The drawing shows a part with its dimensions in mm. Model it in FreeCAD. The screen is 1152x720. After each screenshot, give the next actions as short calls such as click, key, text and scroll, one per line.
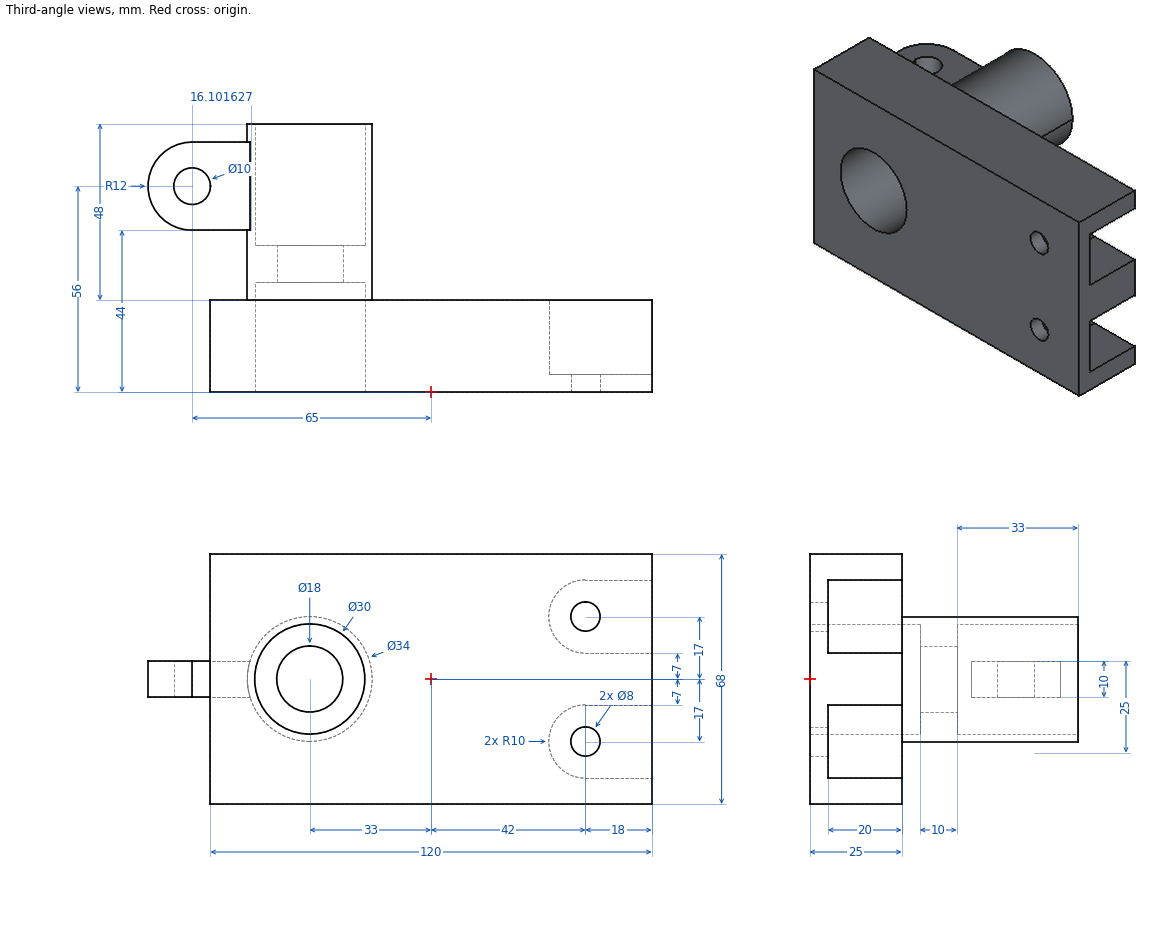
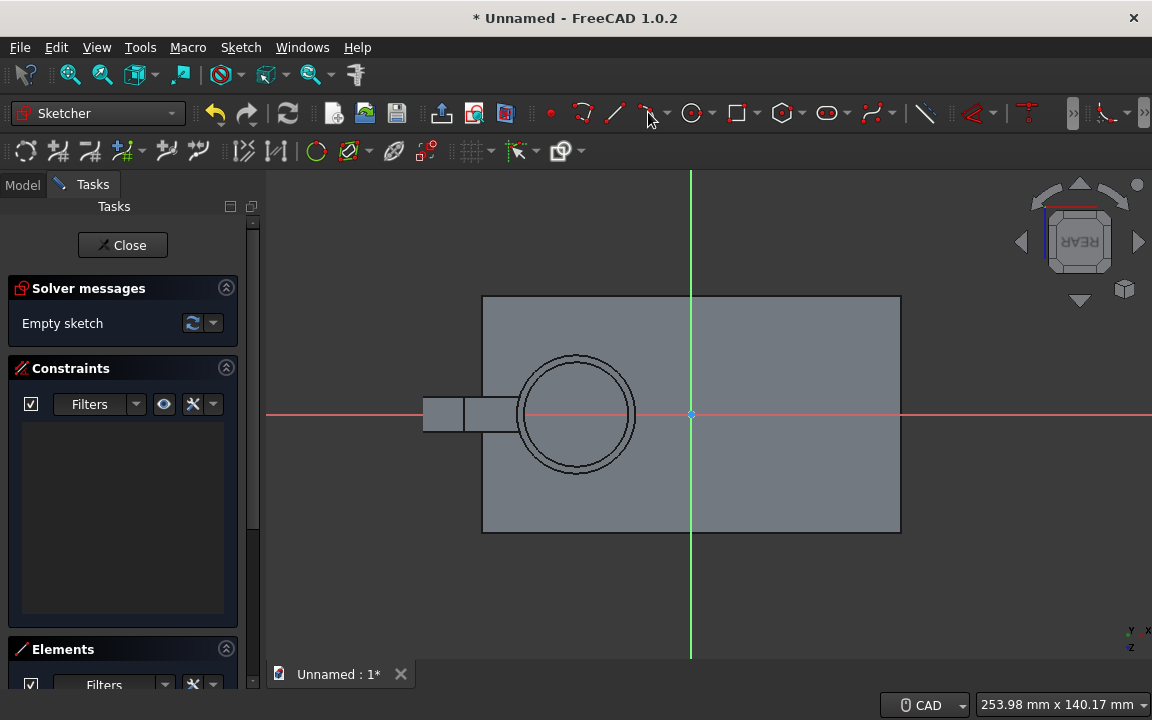
scroll(608, 414, up, 6)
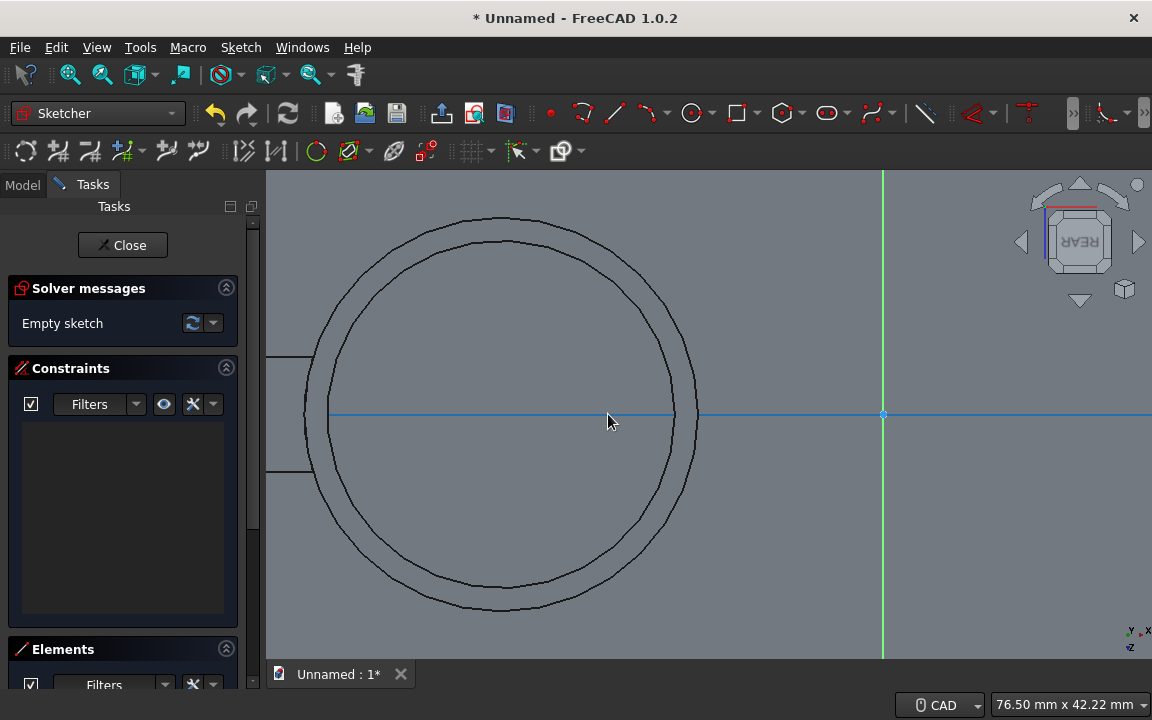
click(692, 114)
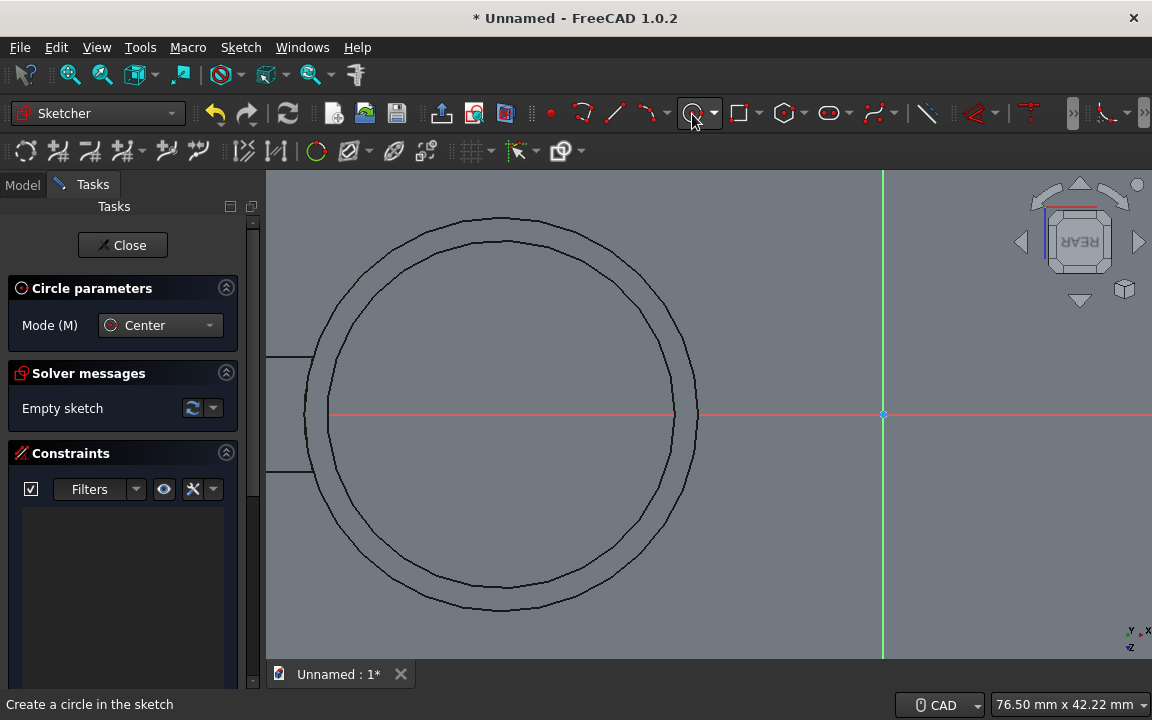
click(501, 414)
move(575, 341)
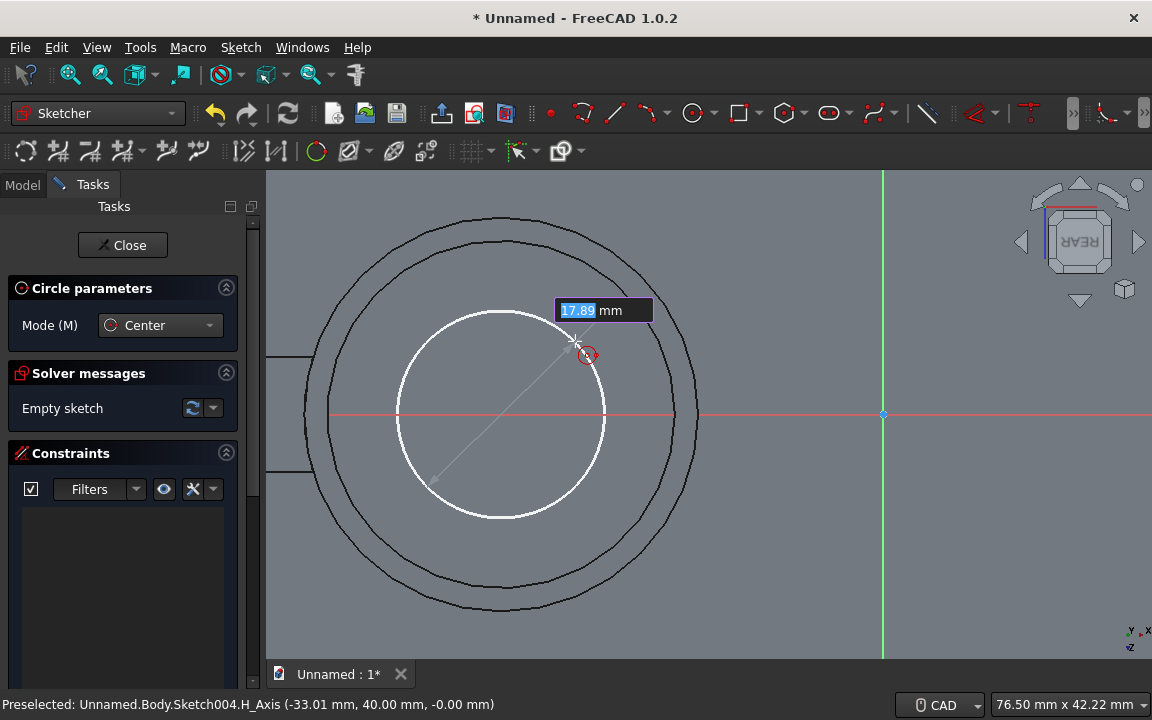
text(18)
key(Return)
key(Escape)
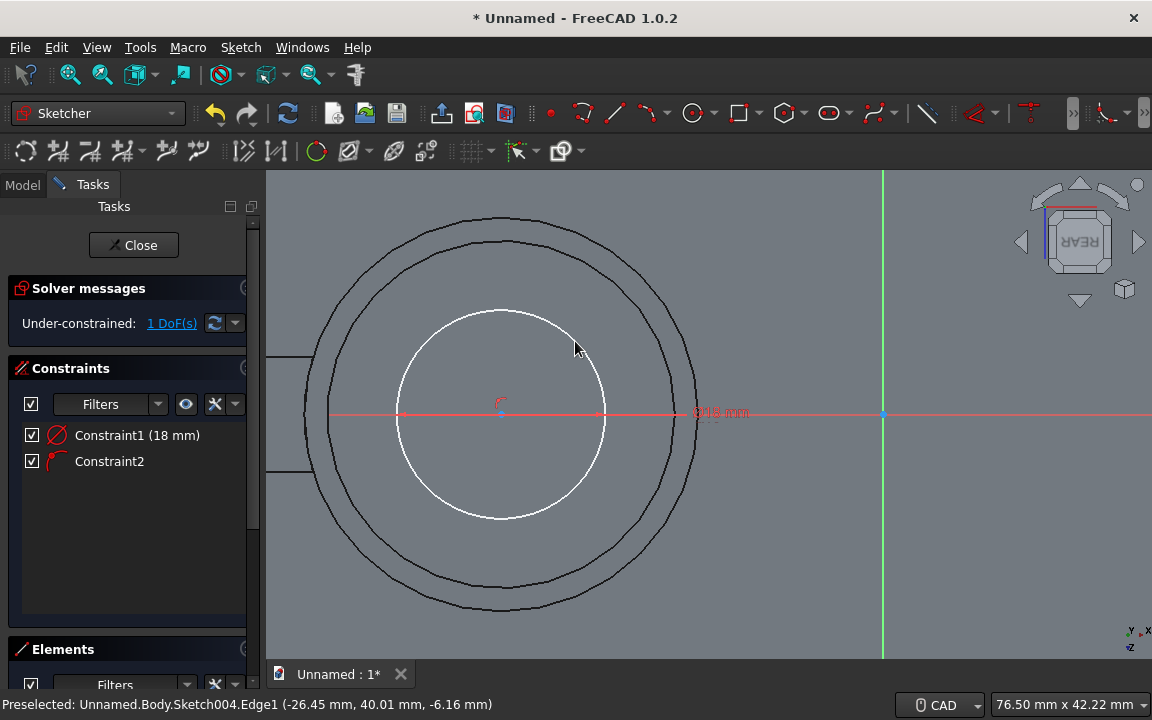
click(974, 114)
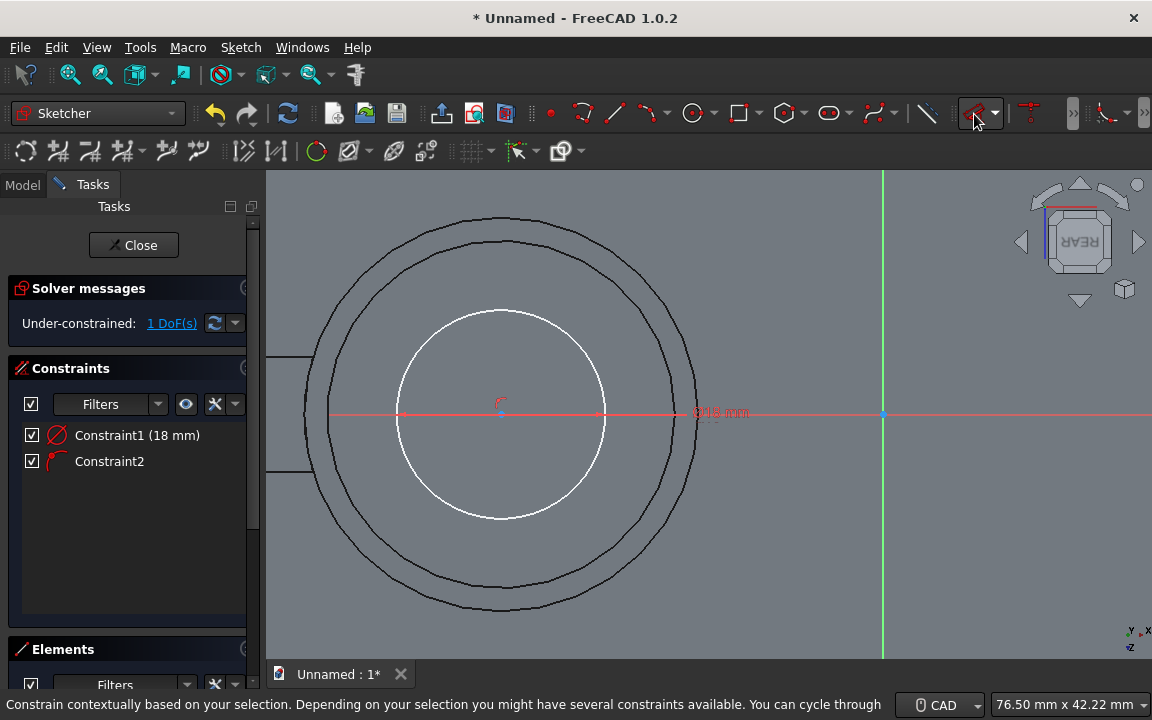
click(501, 414)
click(692, 448)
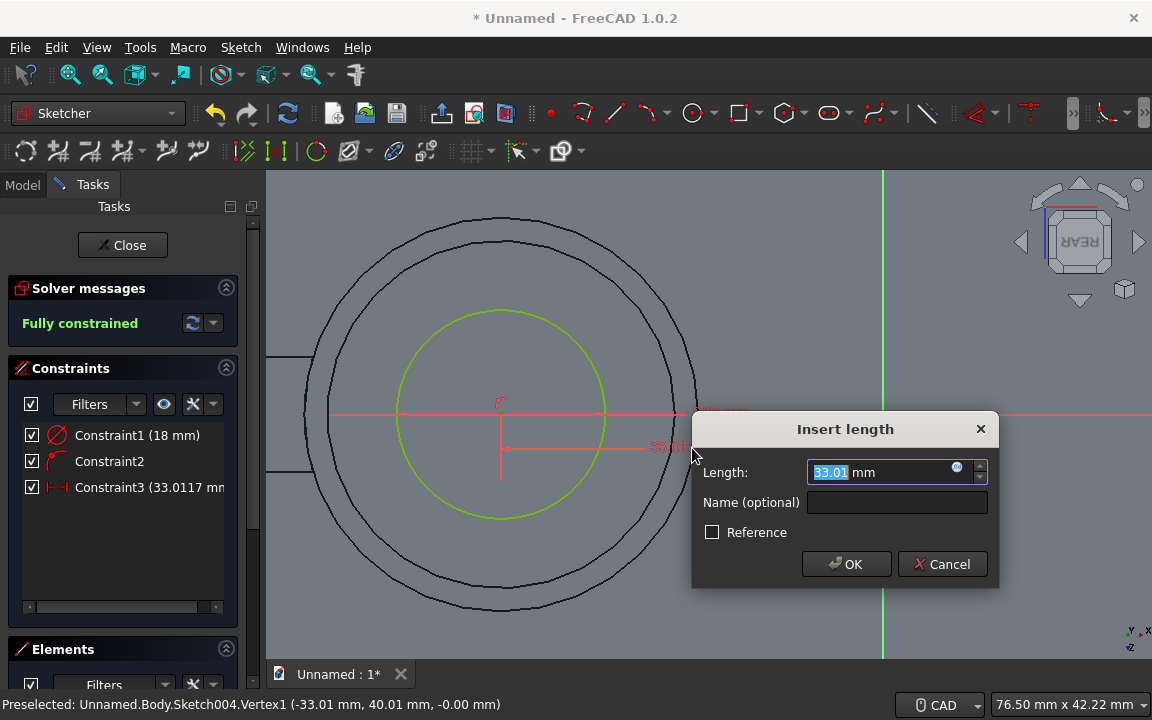
text(33)
key(Return)
key(Escape)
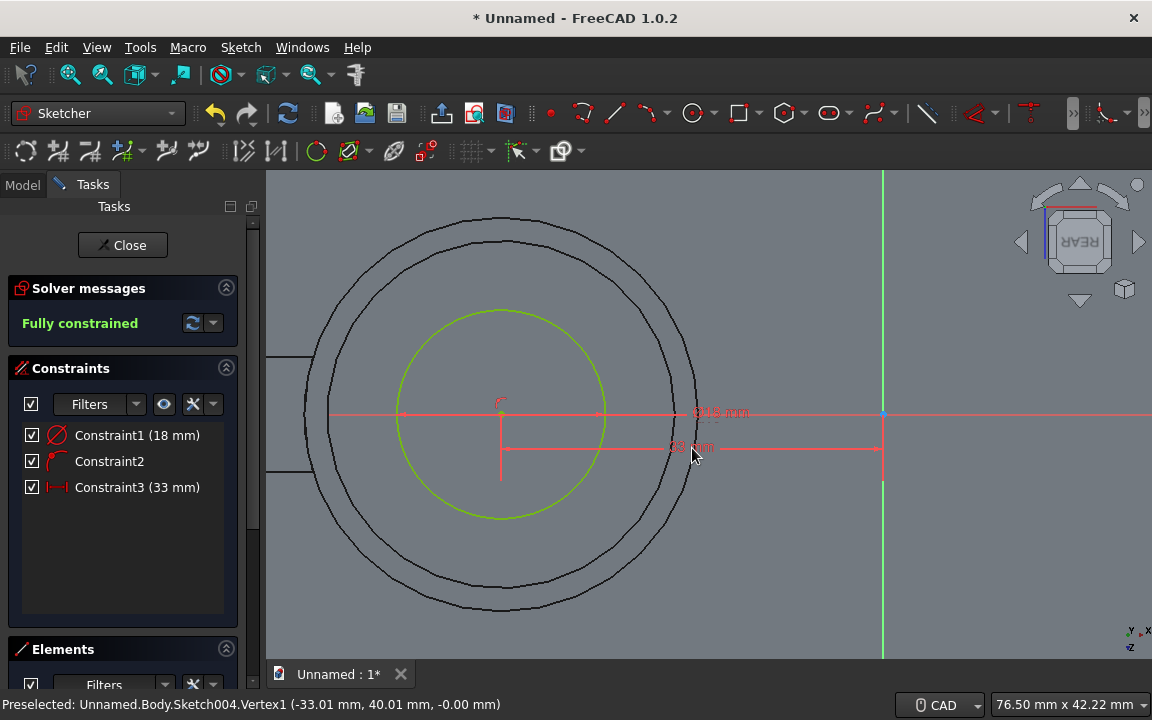
click(123, 245)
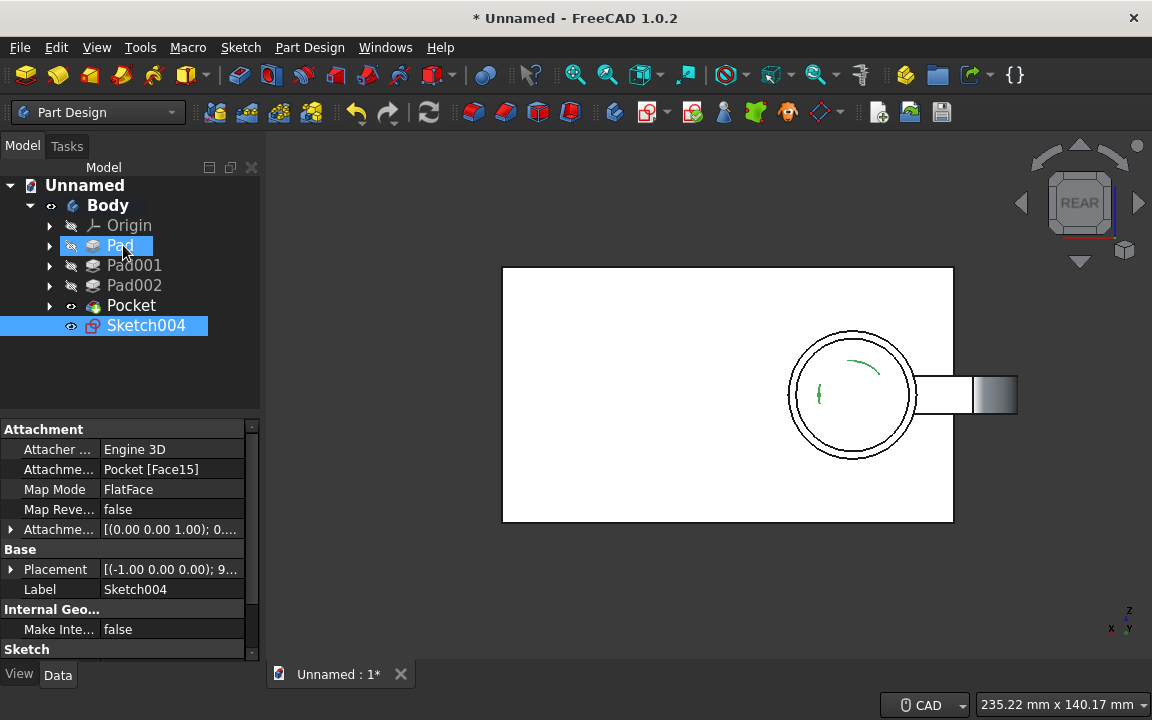
click(240, 76)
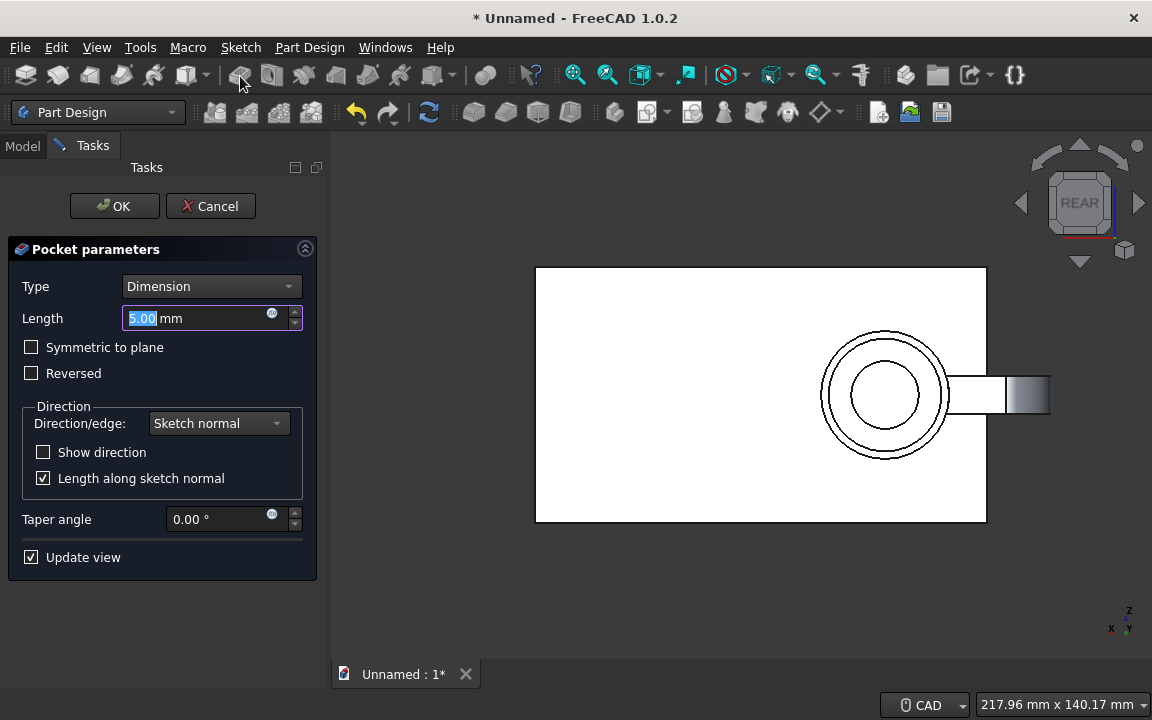
text(10)
key(Tab)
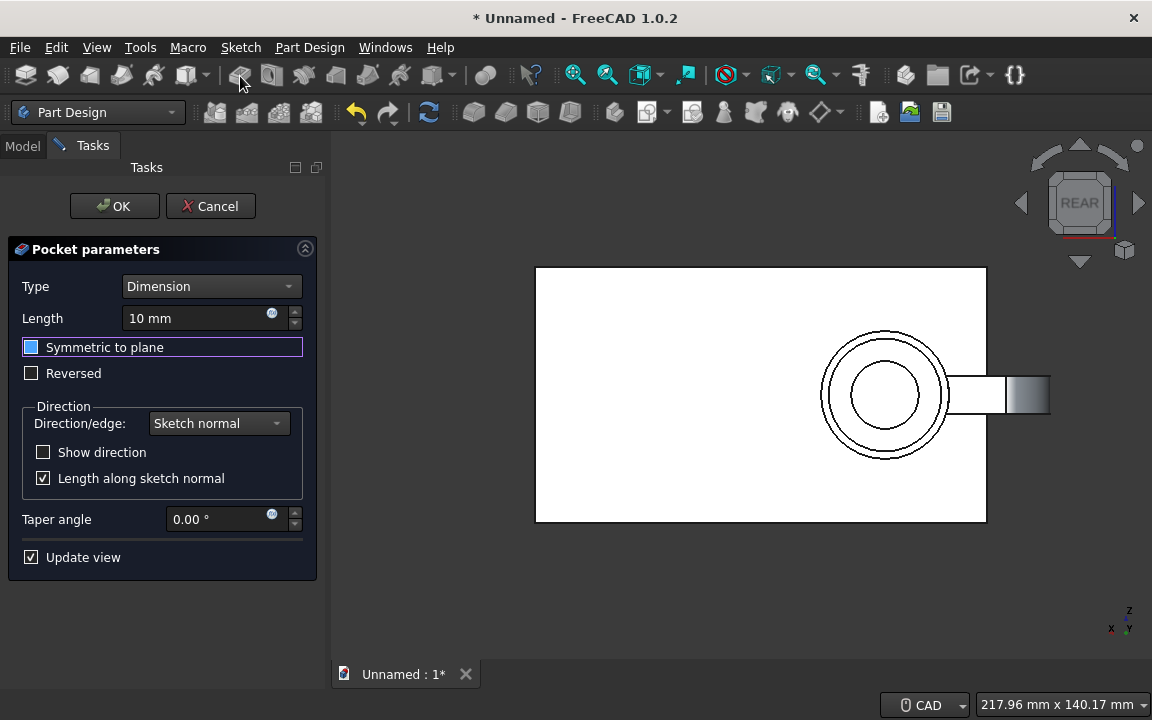
click(115, 206)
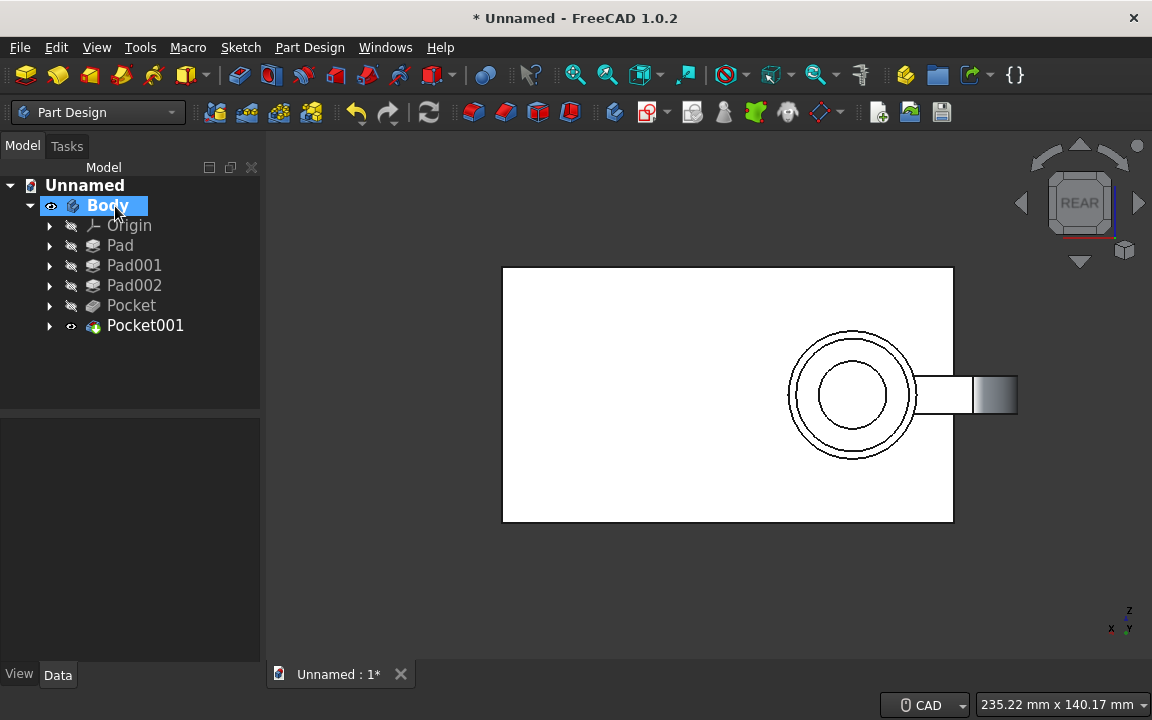
click(853, 394)